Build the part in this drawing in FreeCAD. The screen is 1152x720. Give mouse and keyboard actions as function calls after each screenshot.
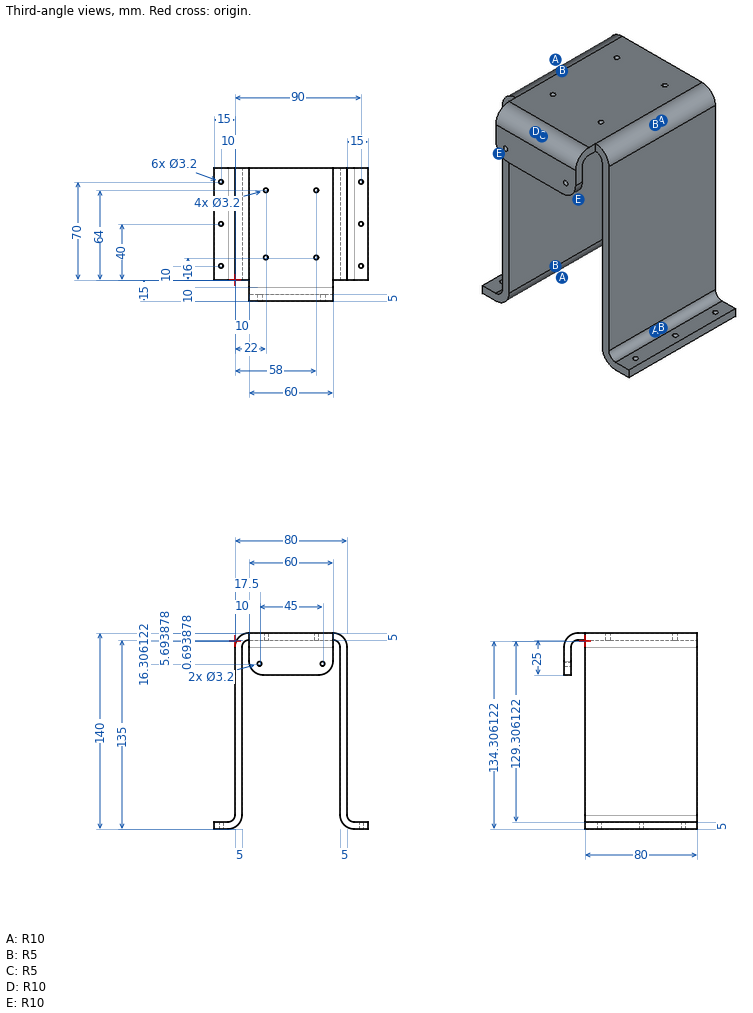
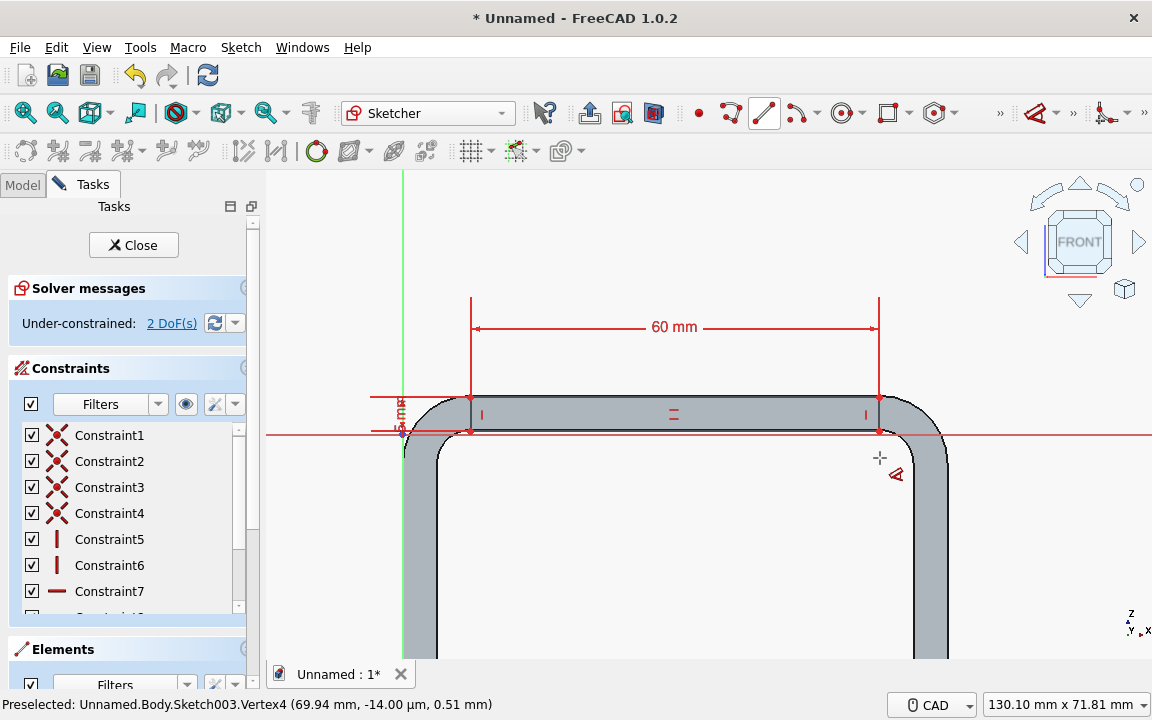
click(471, 397)
click(437, 469)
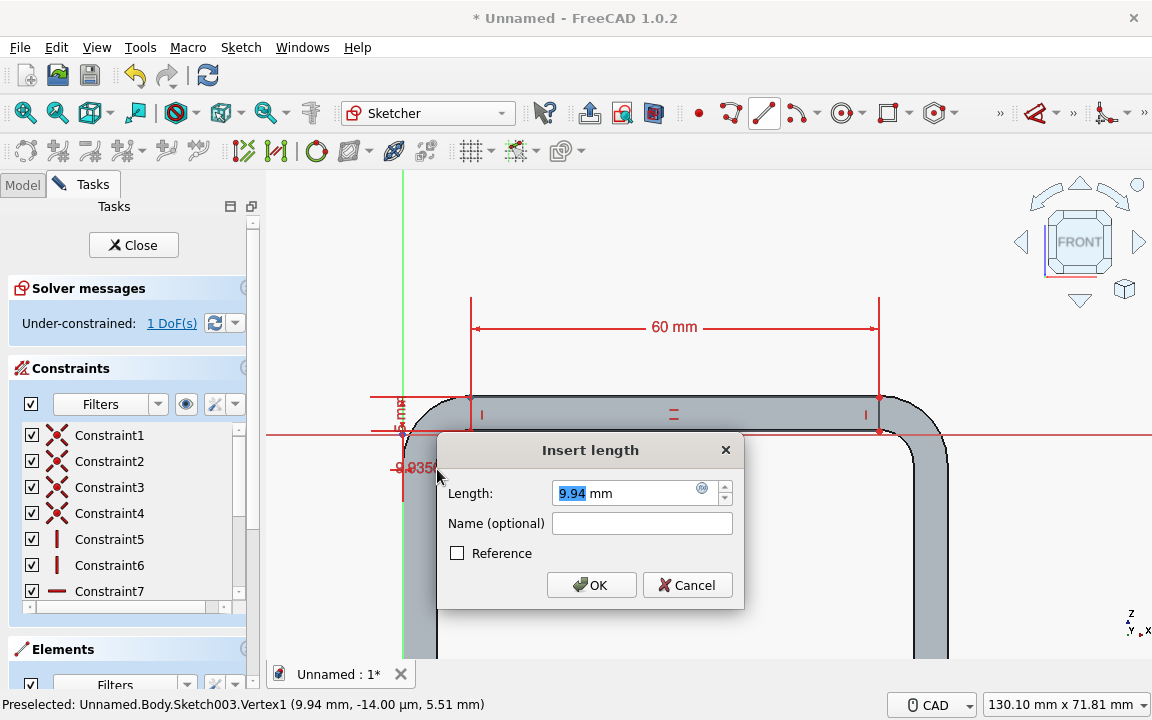
text(10)
key(Return)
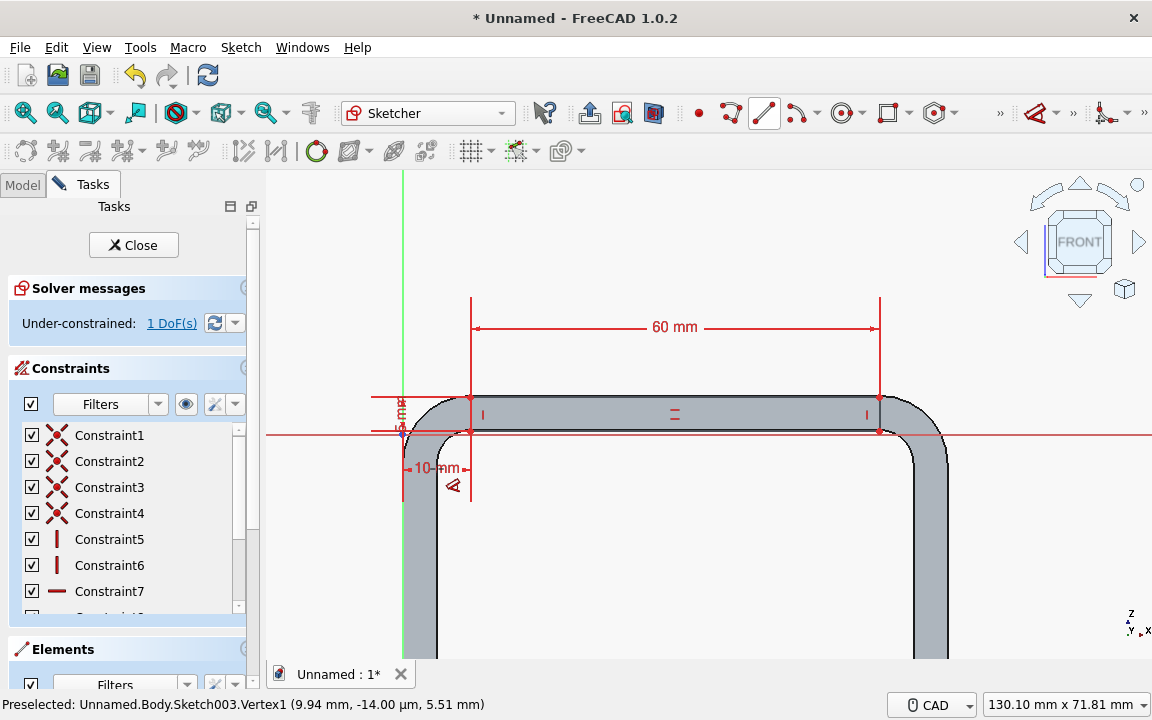
click(471, 397)
click(369, 416)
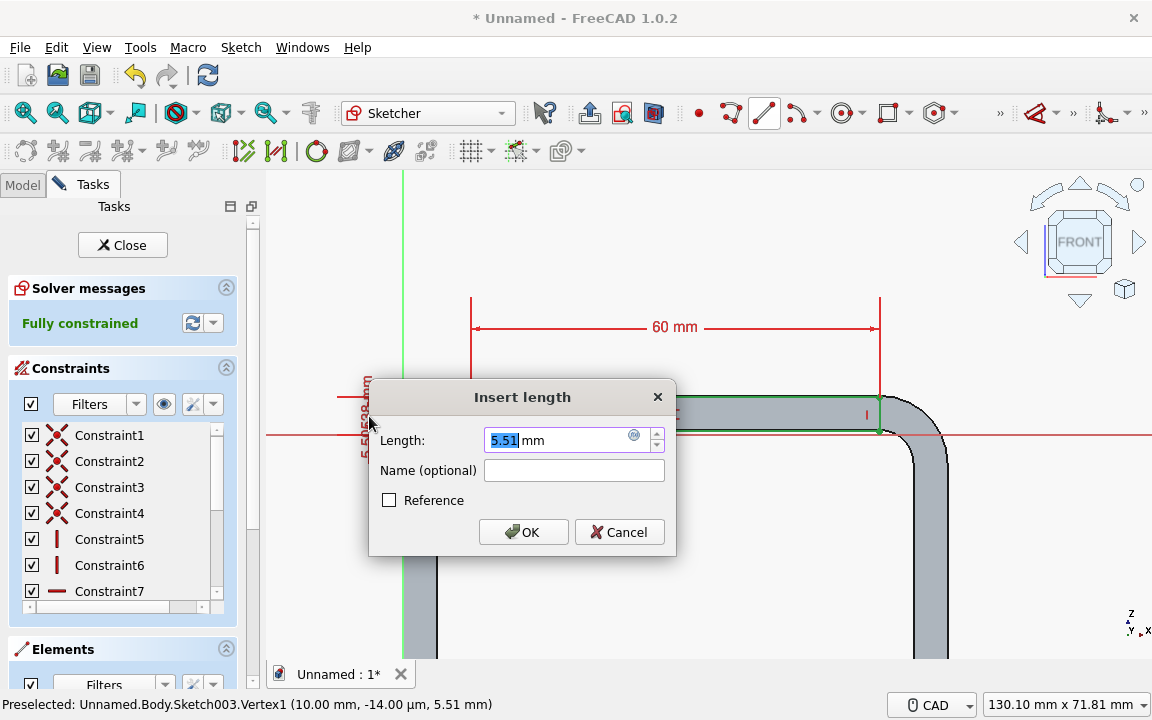
text(5.693878)
key(Return)
key(Escape)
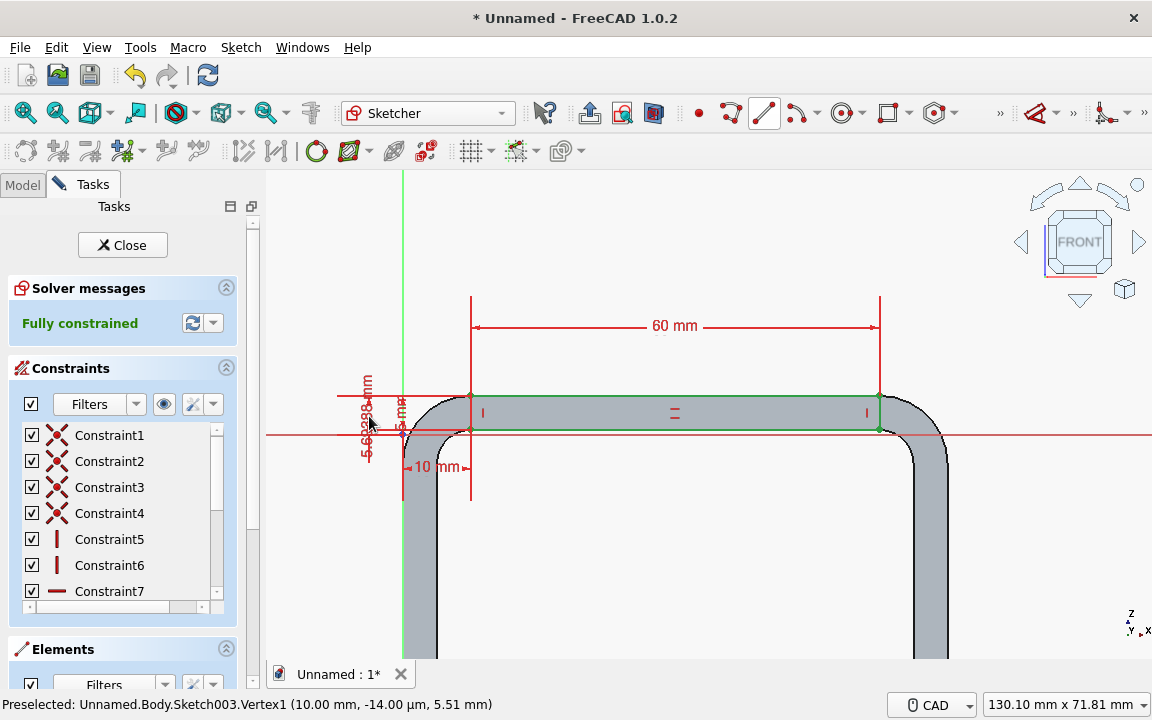
click(123, 245)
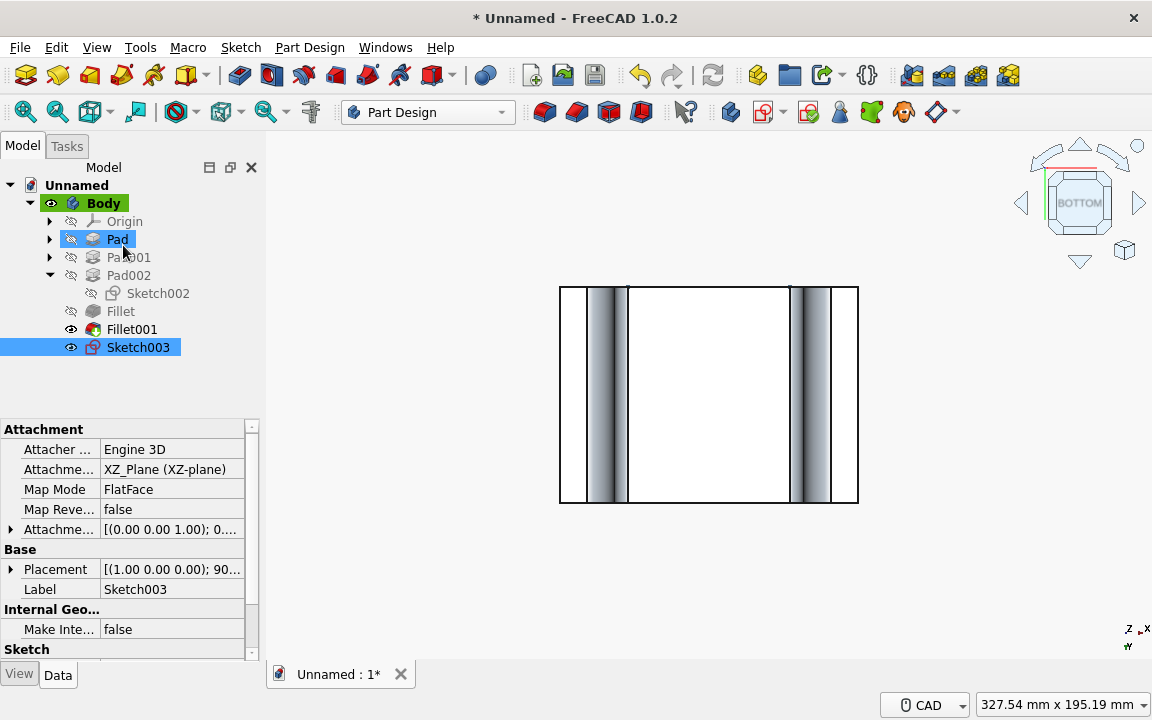
click(26, 76)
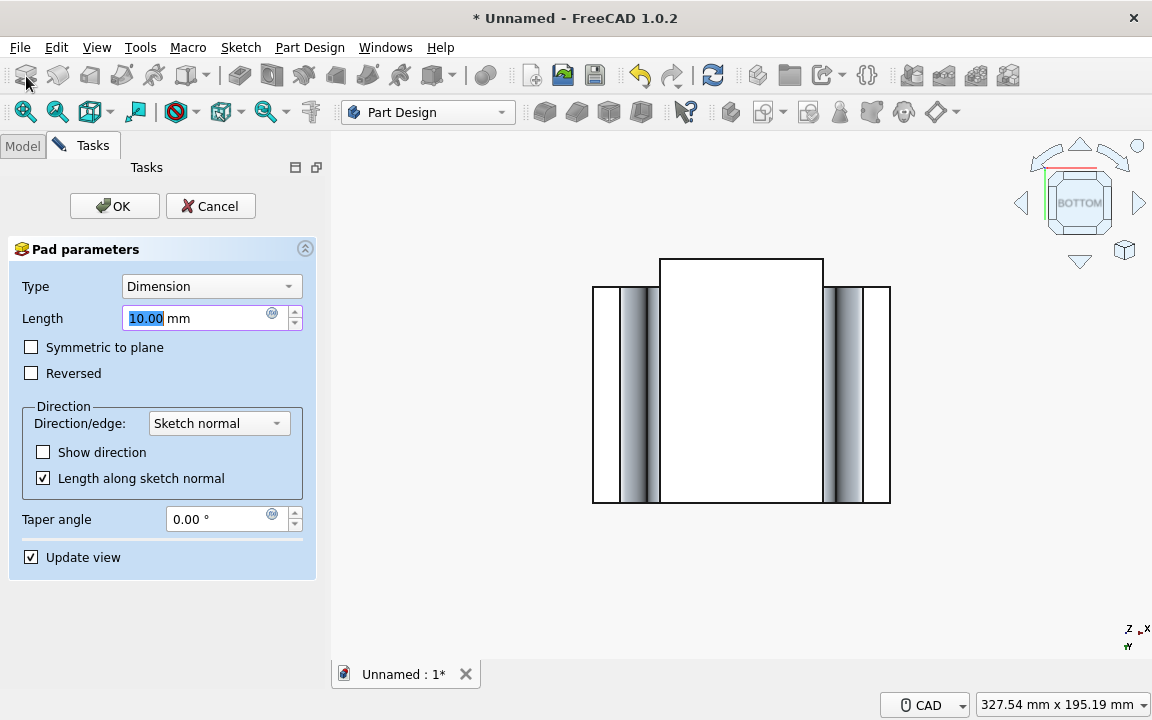
text(15)
key(Tab)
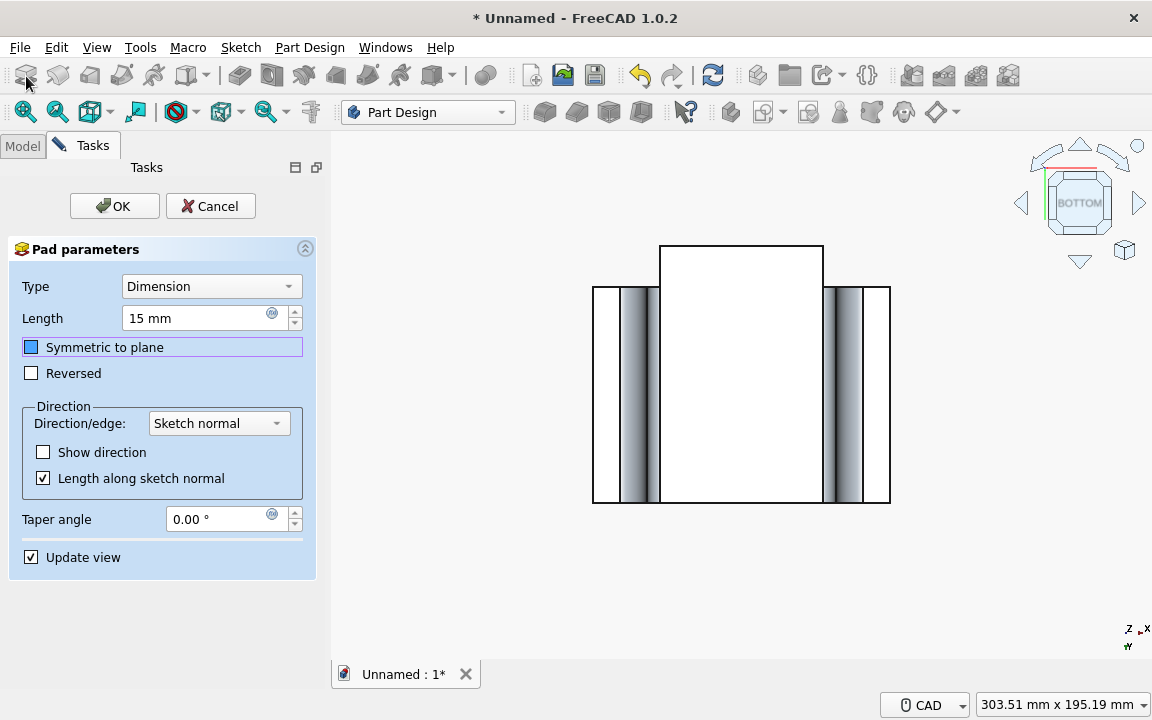
click(115, 206)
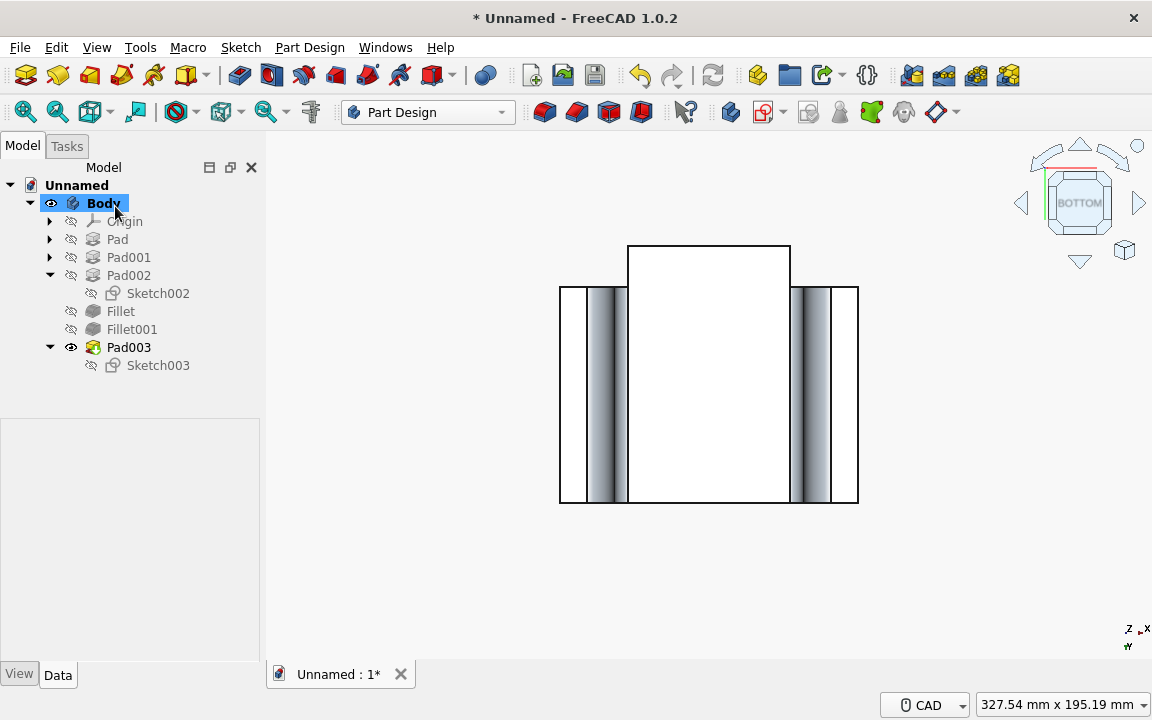
click(709, 410)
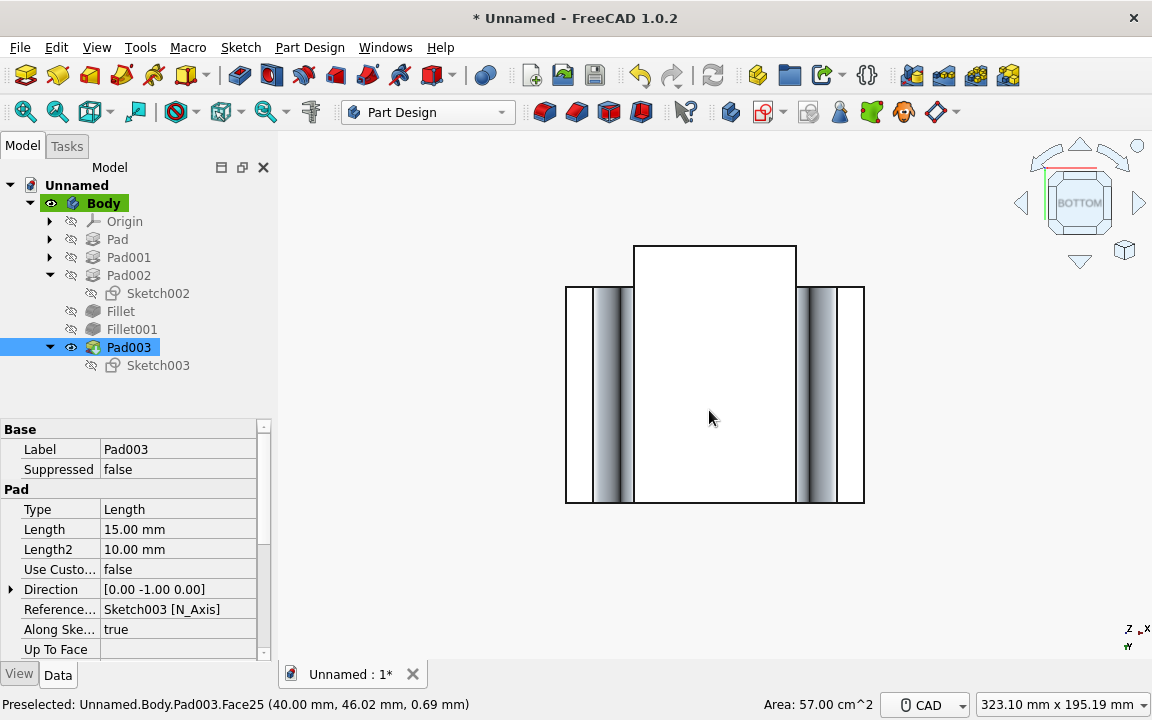
click(764, 112)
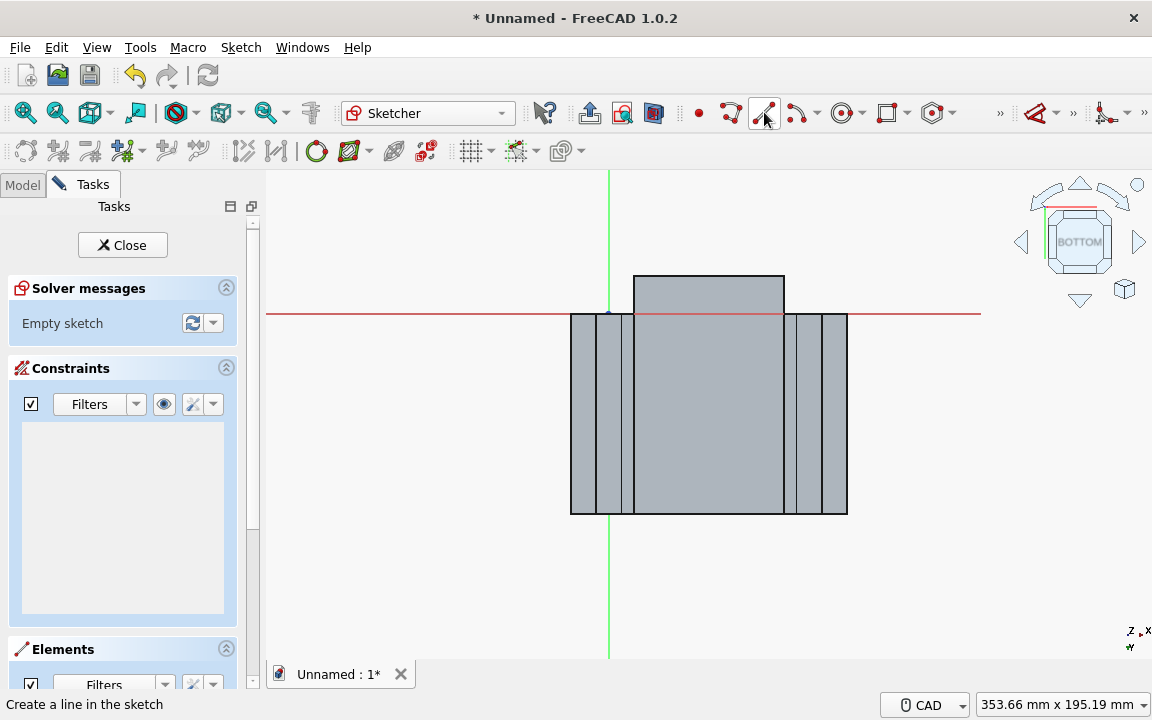
click(654, 114)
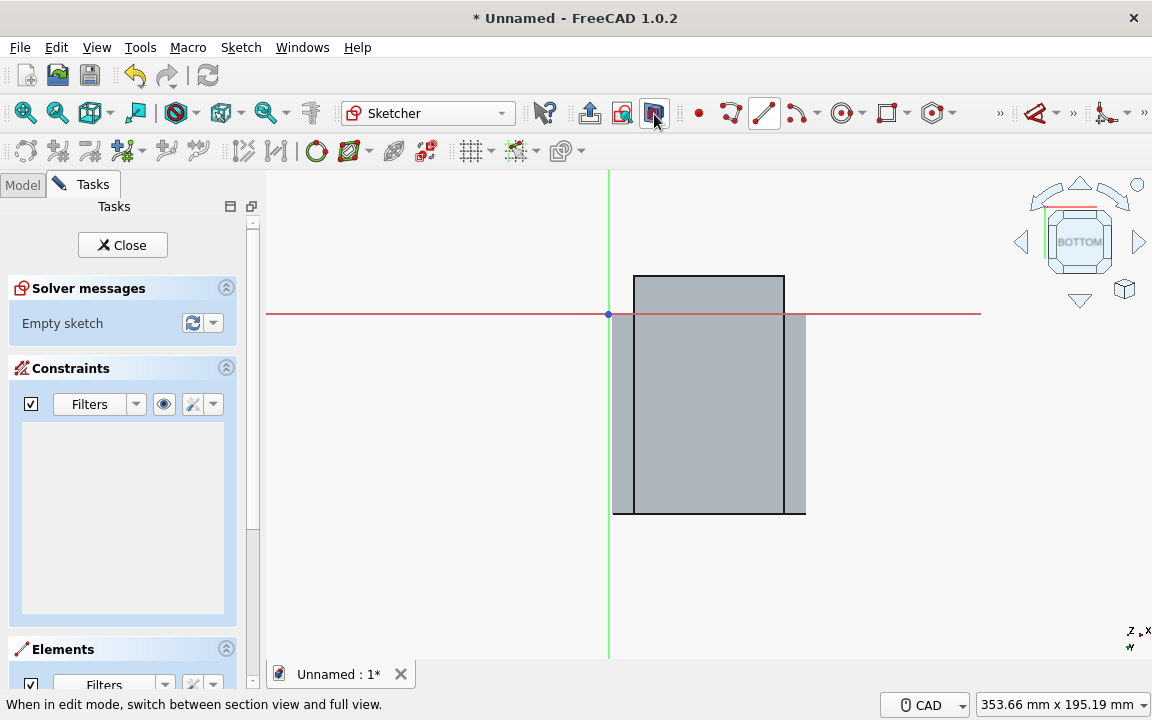
scroll(729, 226, up, 5)